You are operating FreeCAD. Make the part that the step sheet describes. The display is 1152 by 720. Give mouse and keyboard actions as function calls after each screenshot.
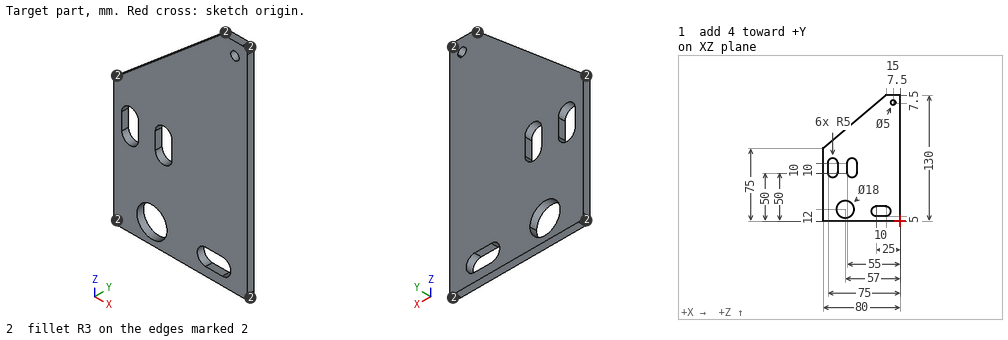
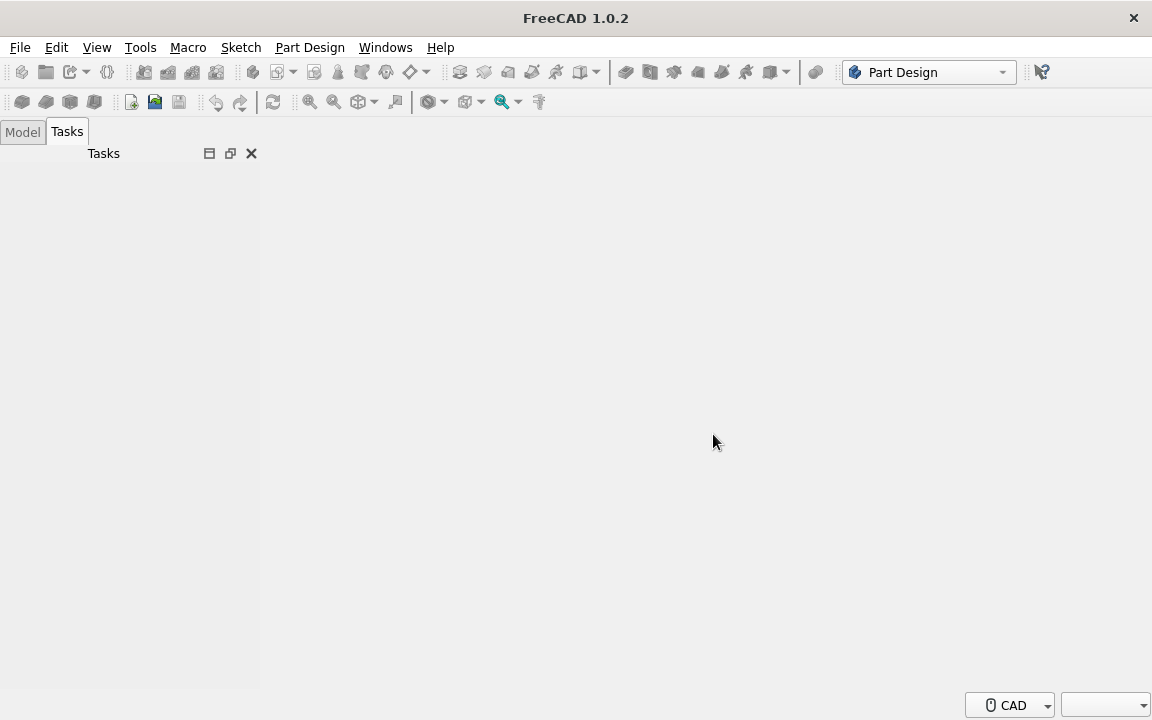
click(132, 102)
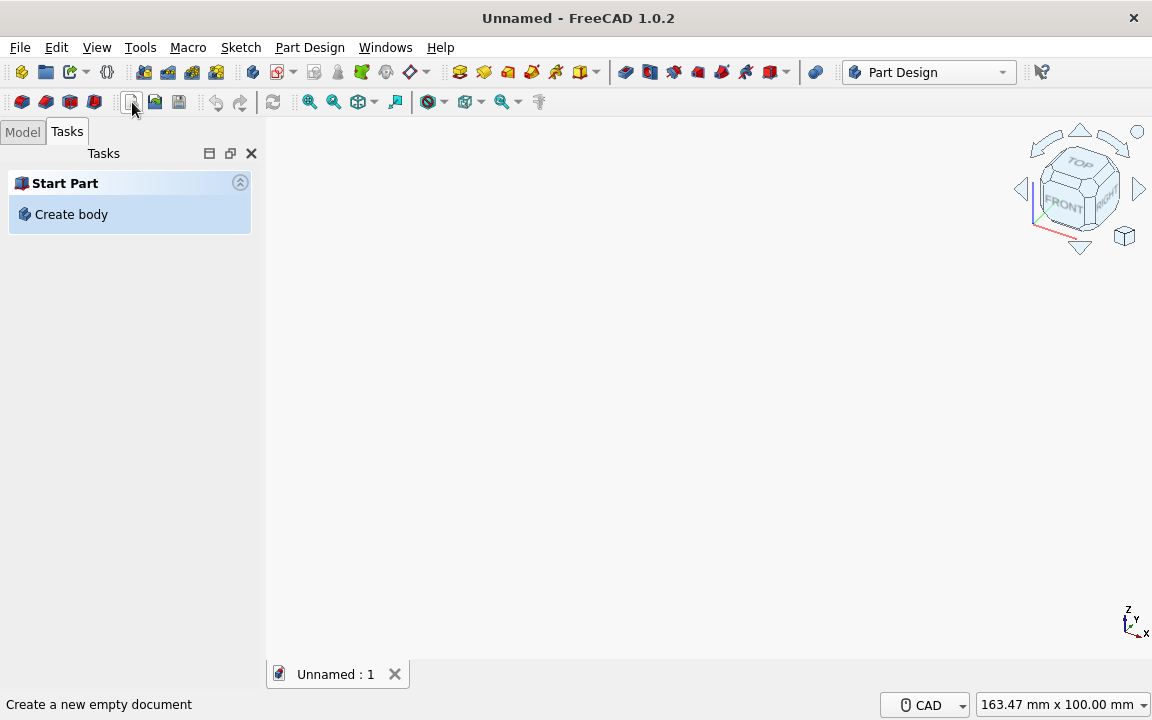
click(278, 72)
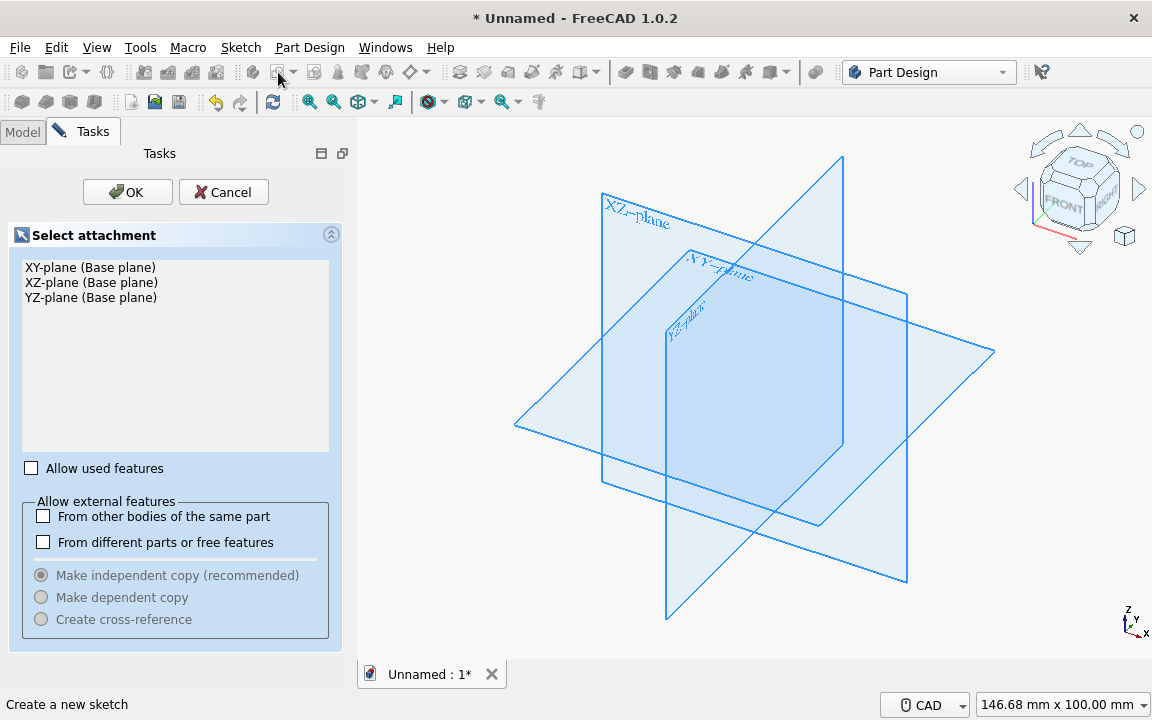
click(82, 282)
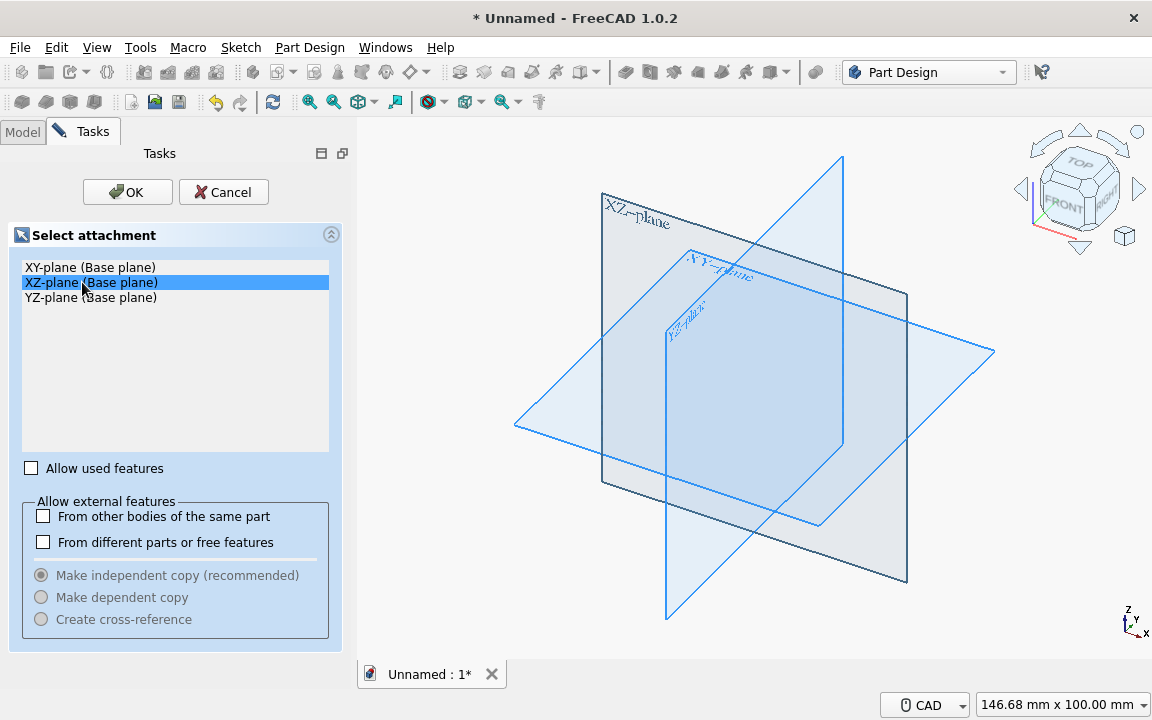
click(128, 192)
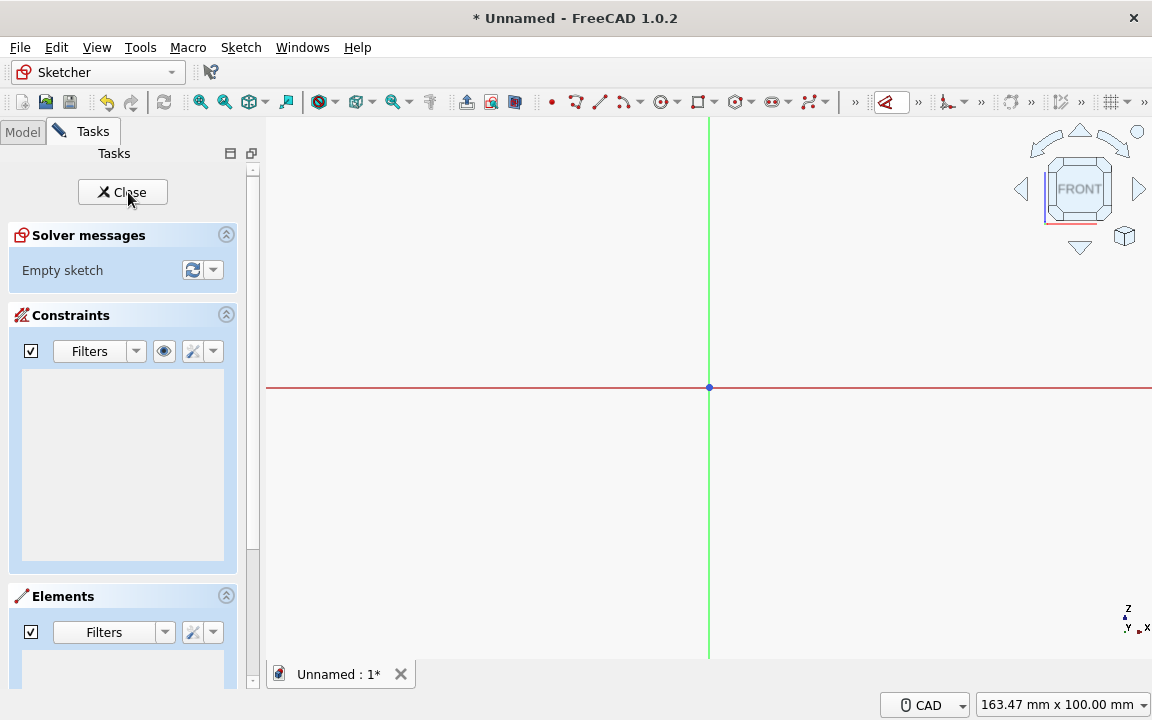
scroll(762, 631, down, 4)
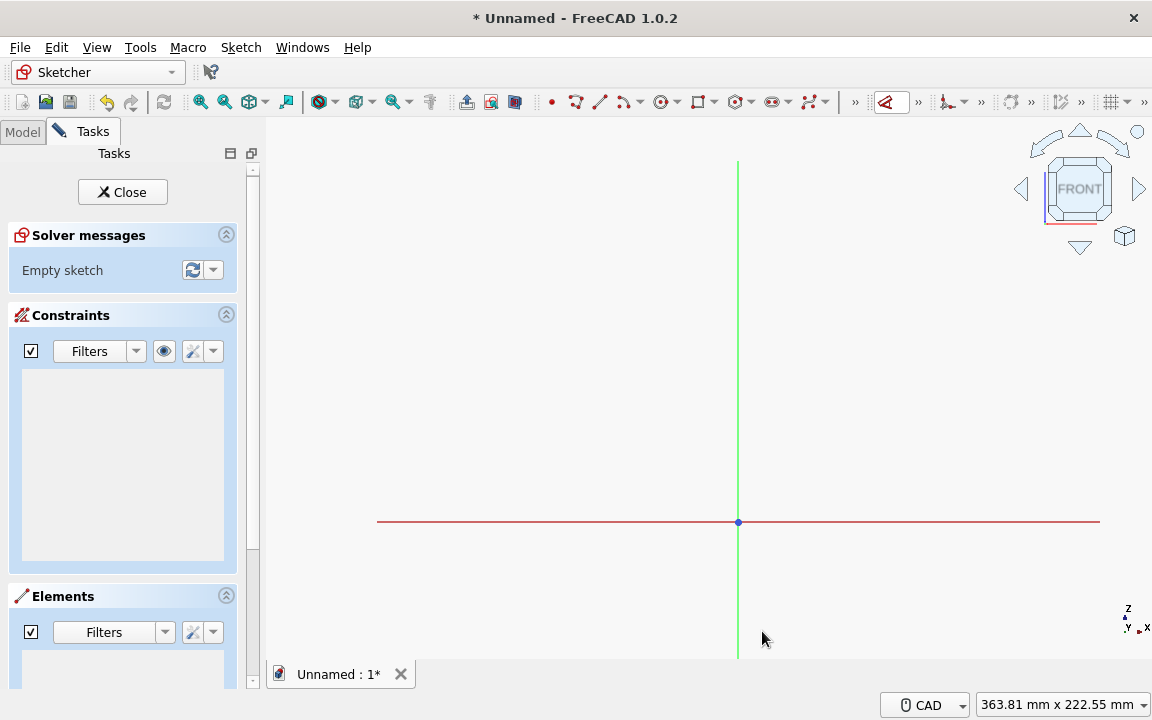
click(576, 102)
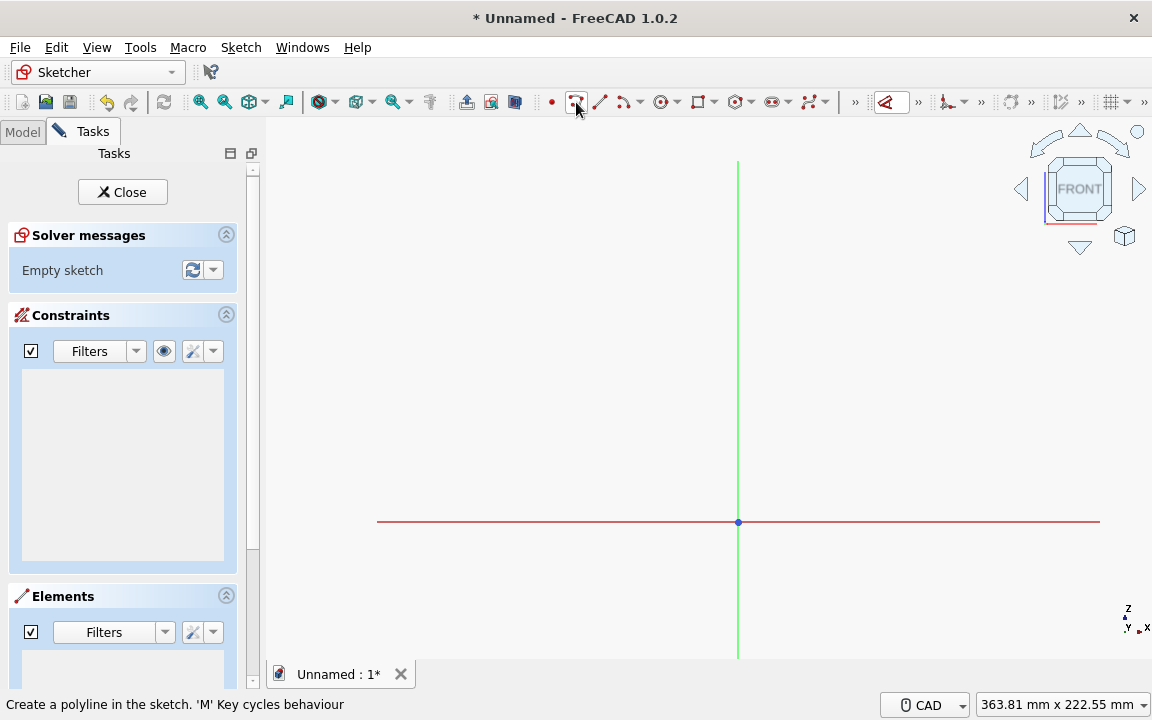
click(738, 522)
click(544, 513)
click(544, 340)
click(702, 206)
click(729, 206)
click(738, 522)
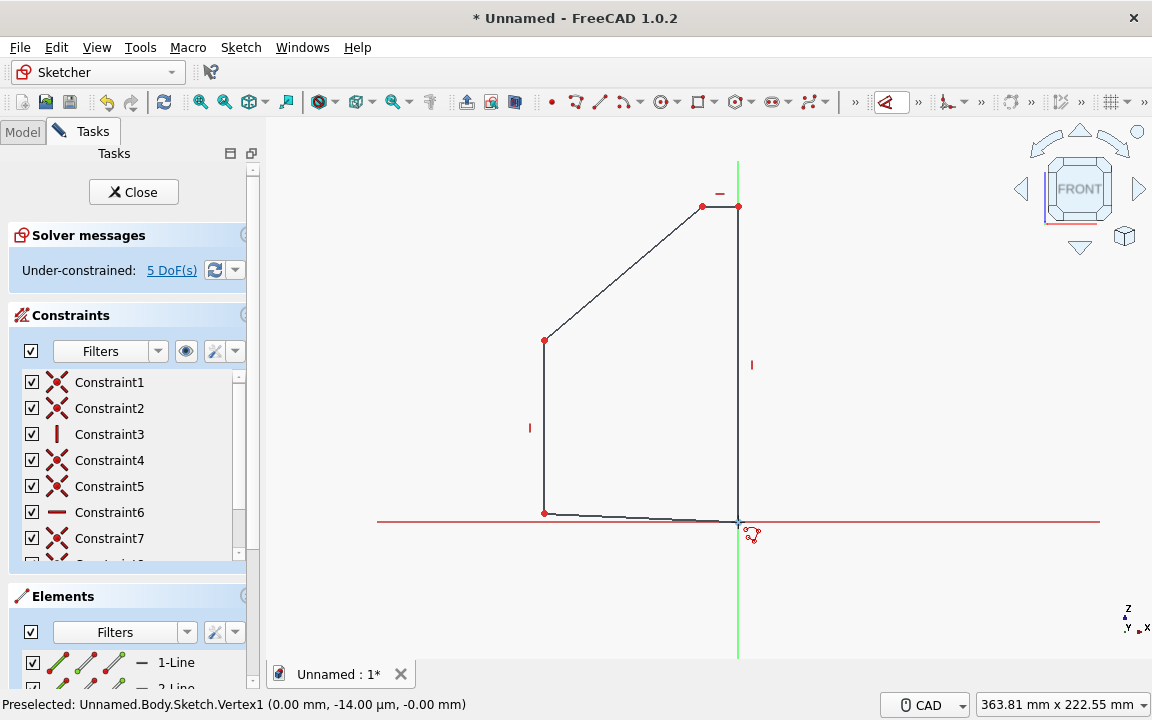
click(772, 102)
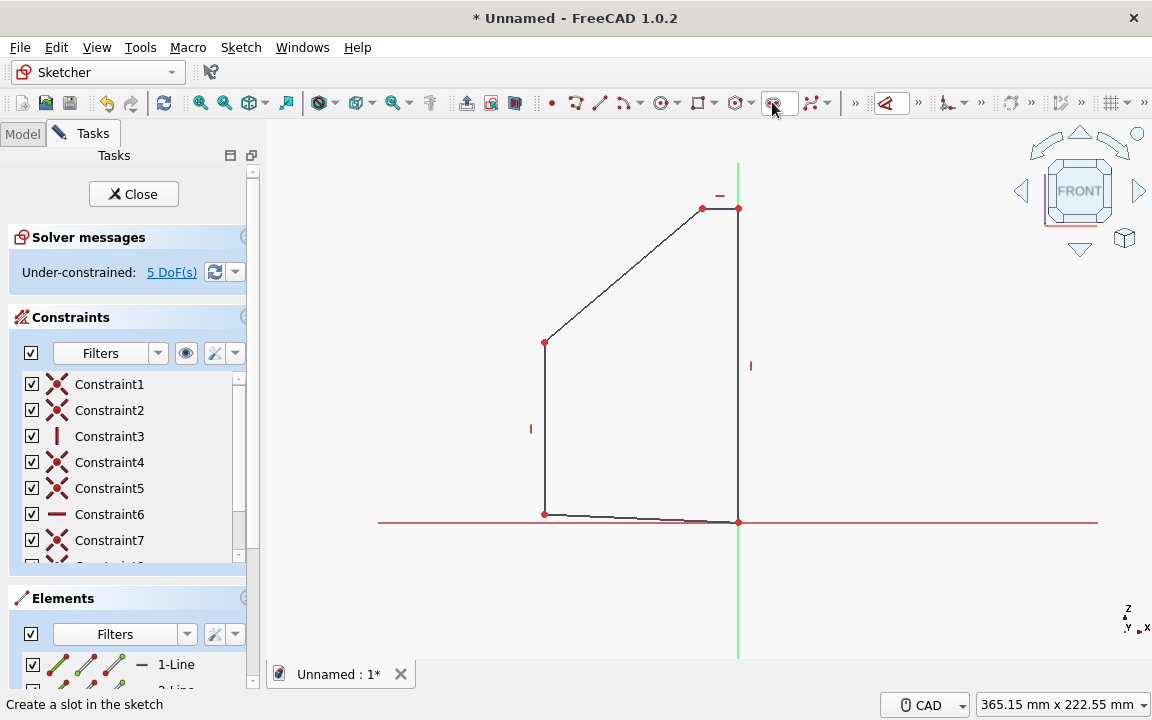
scroll(569, 402, up, 4)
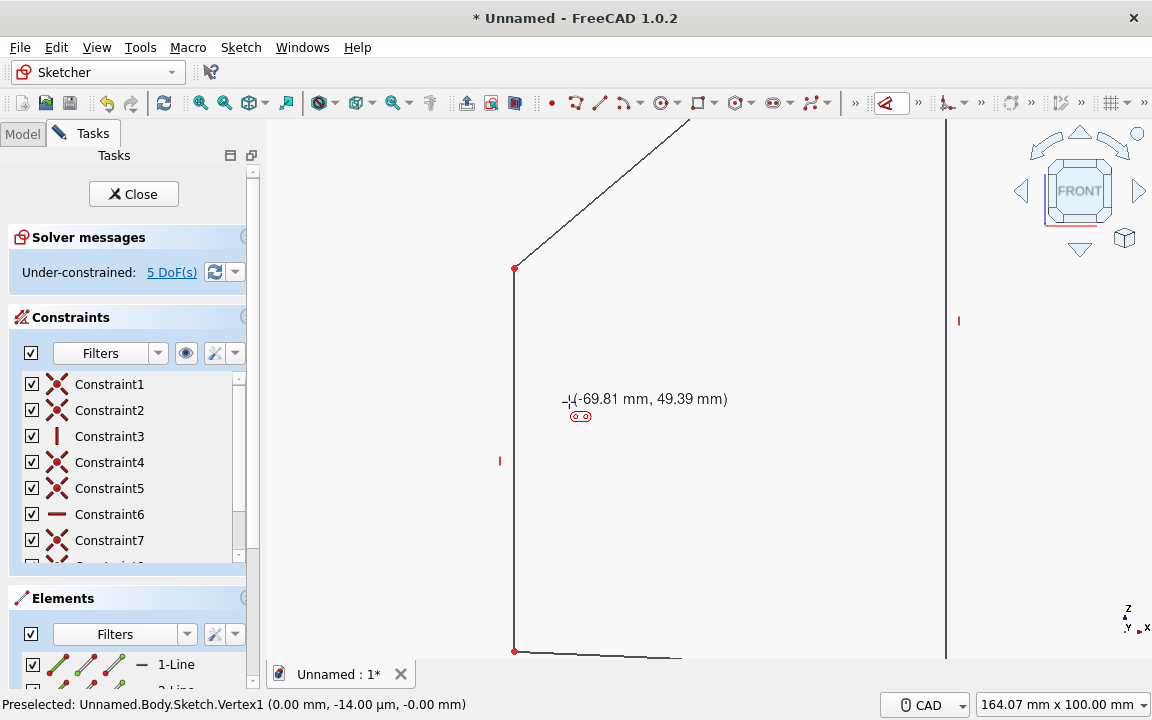
click(568, 400)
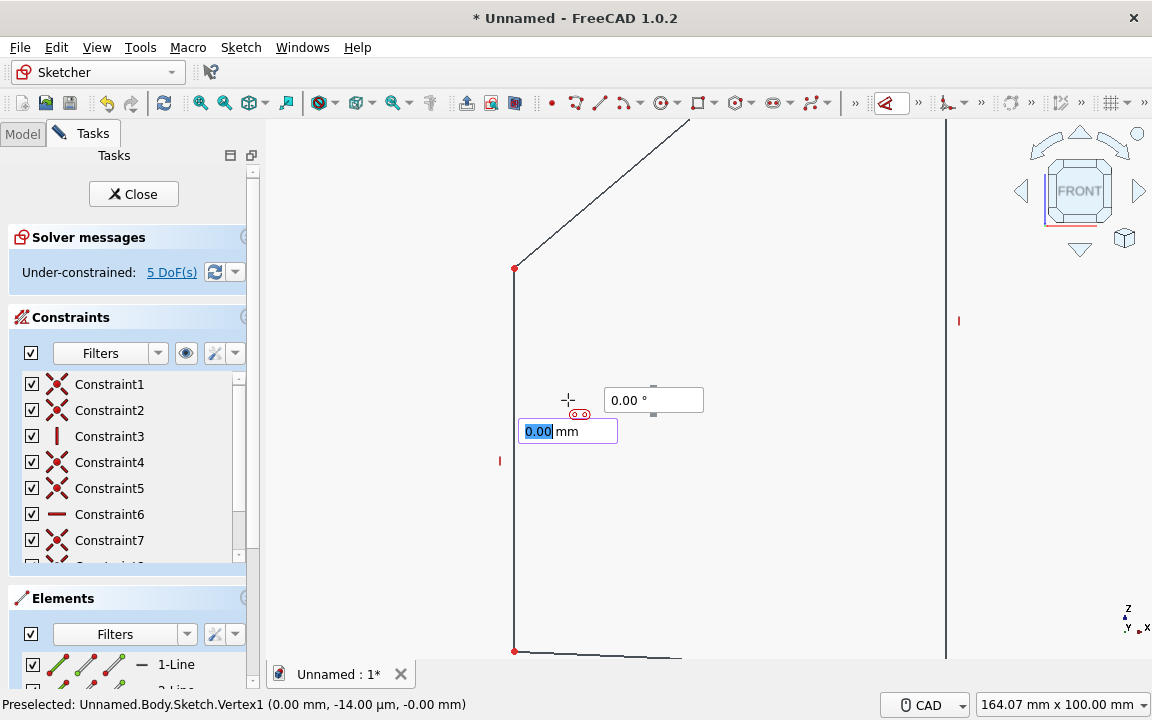
click(568, 346)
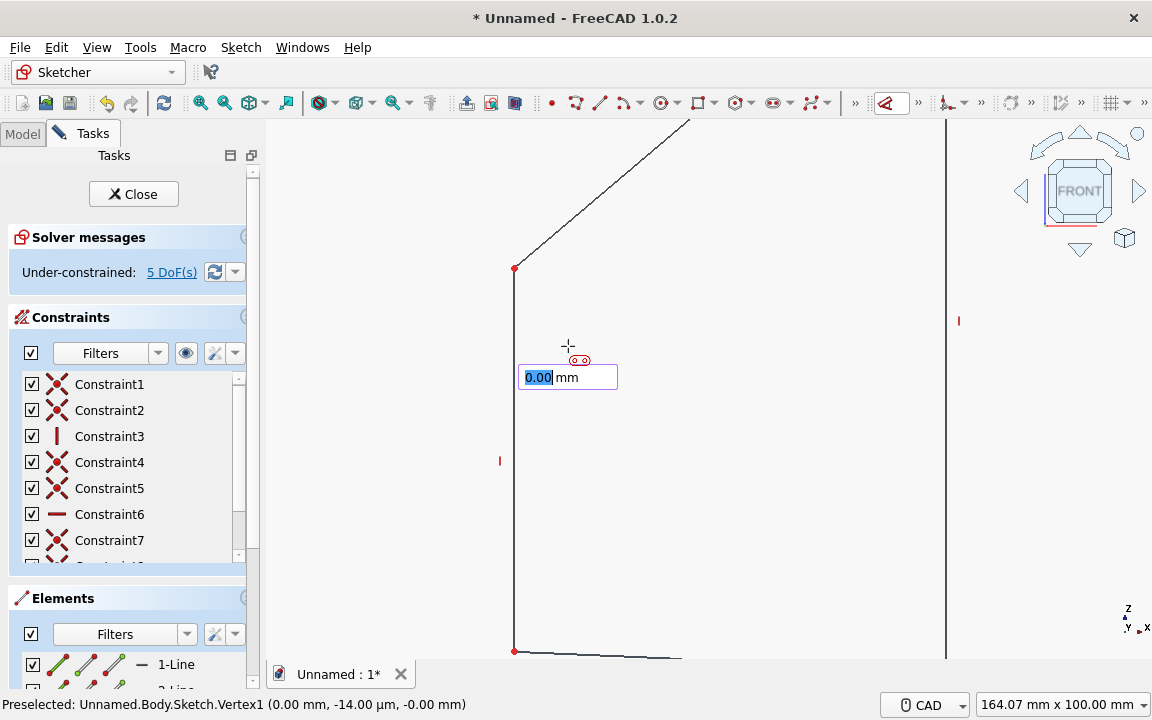
click(595, 373)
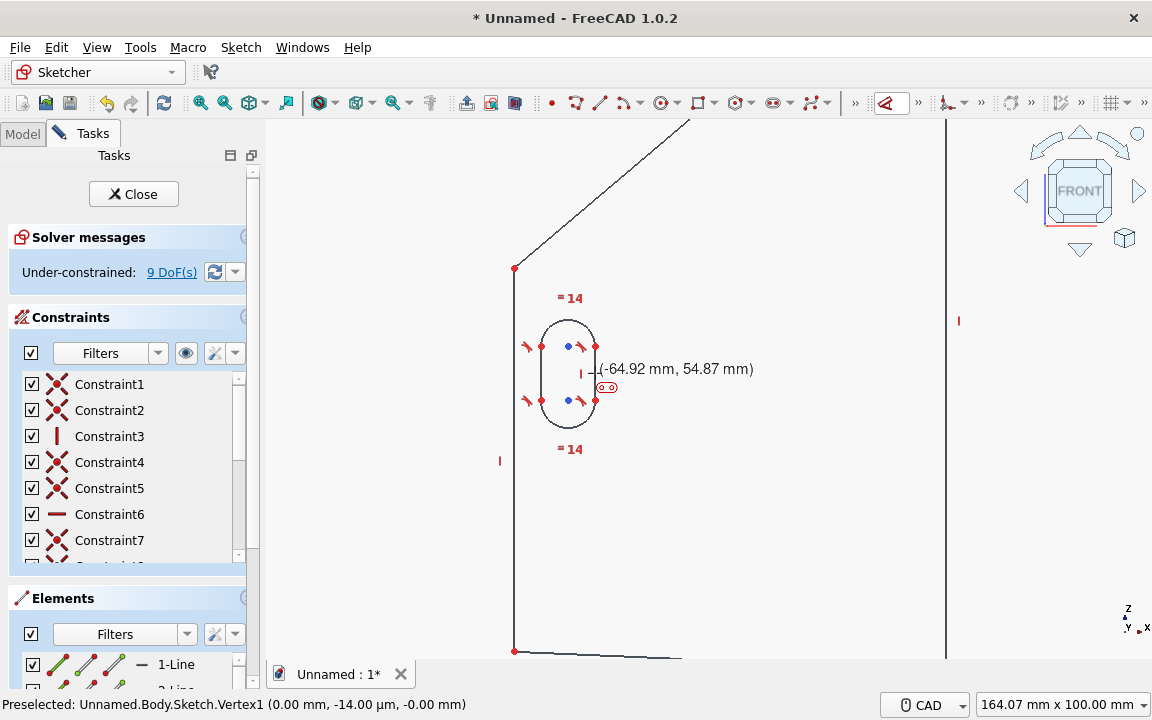
click(676, 400)